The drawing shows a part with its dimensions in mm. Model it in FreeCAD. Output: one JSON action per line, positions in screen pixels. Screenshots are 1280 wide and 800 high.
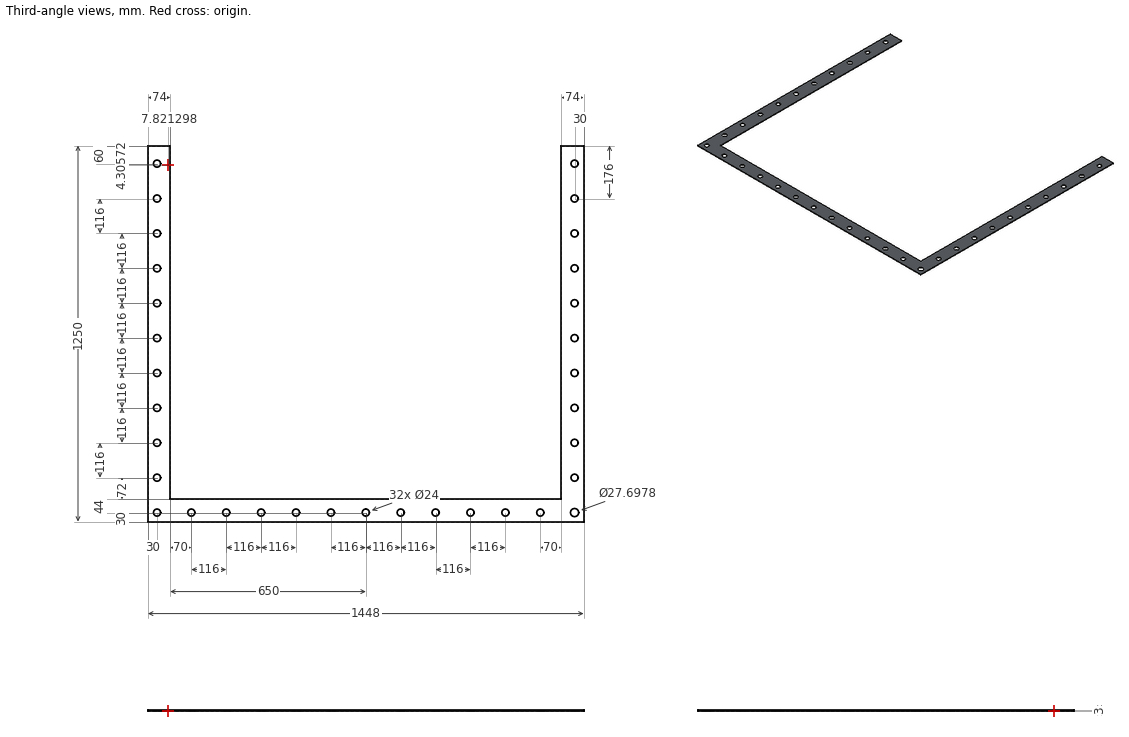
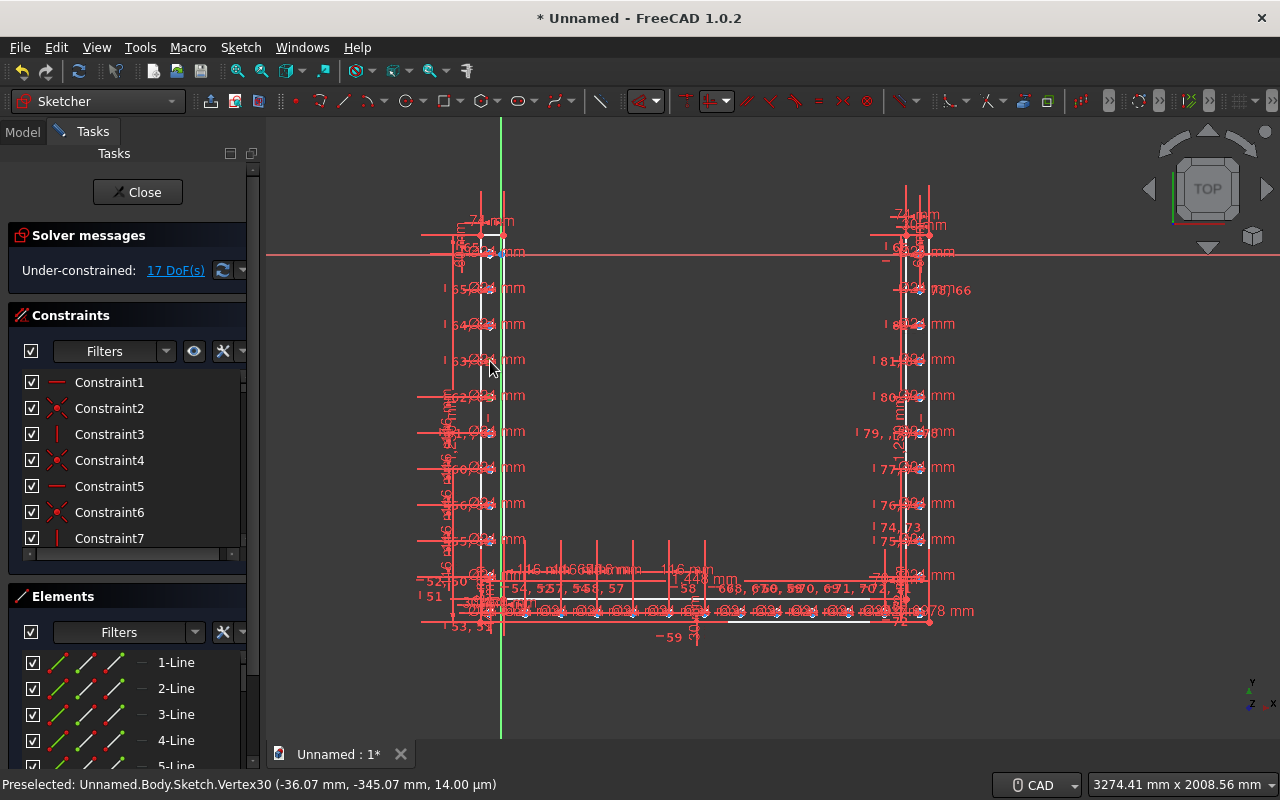
{"action": "left_click", "coordinate": [658, 102]}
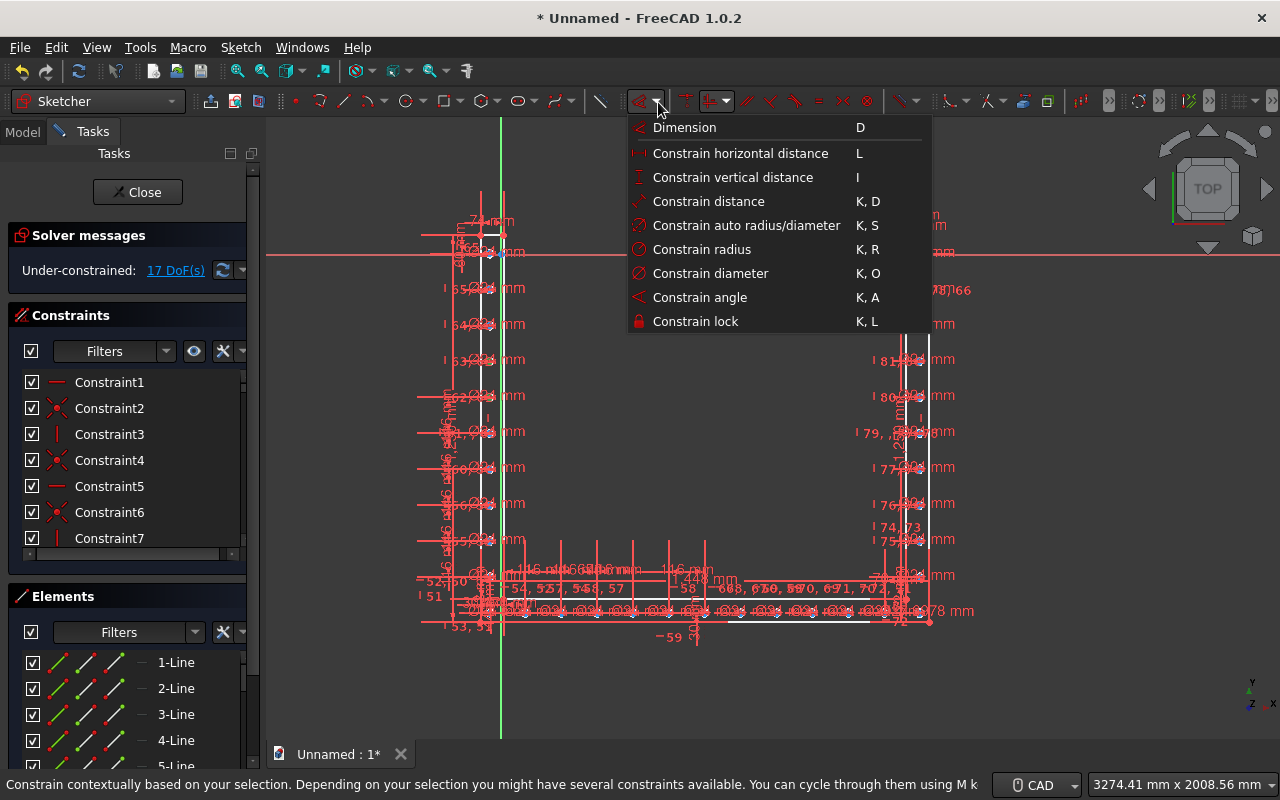
{"action": "left_click", "coordinate": [780, 177]}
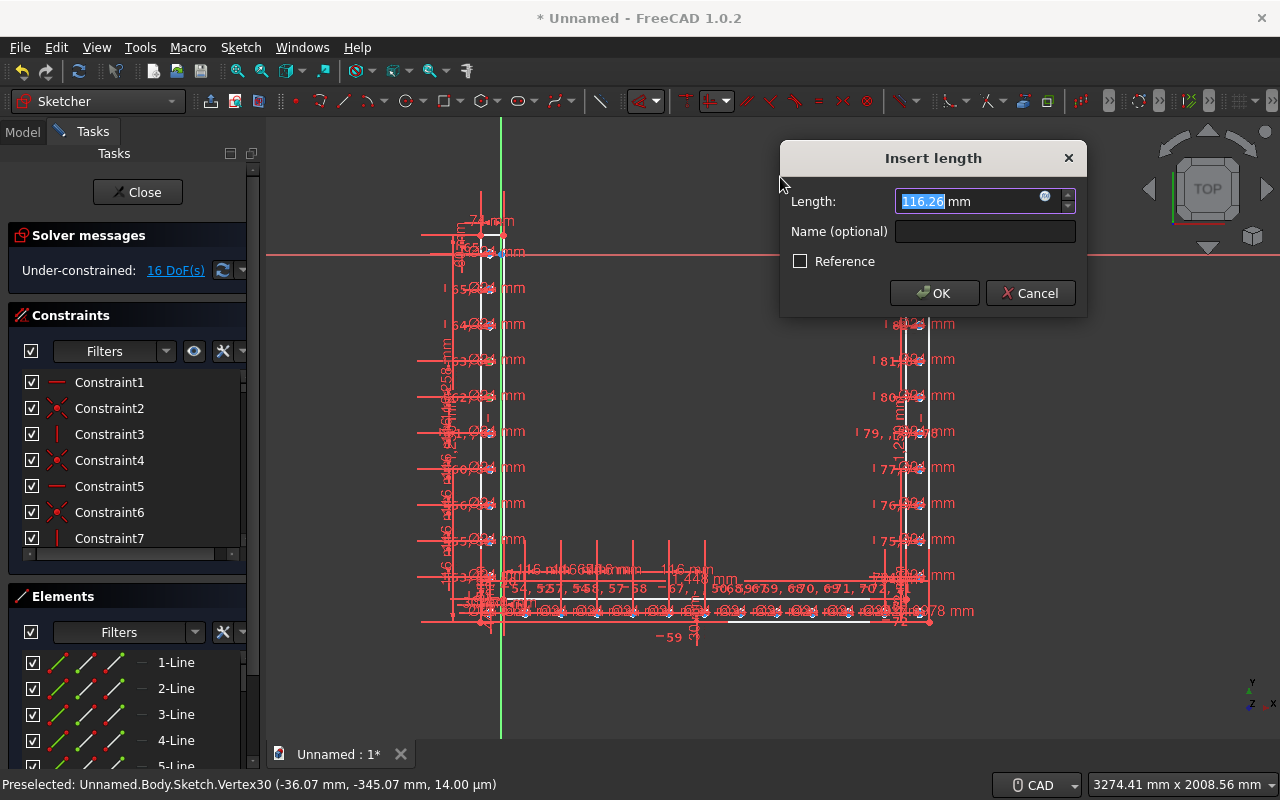
{"action": "type", "text": "116"}
{"action": "key", "text": "Return"}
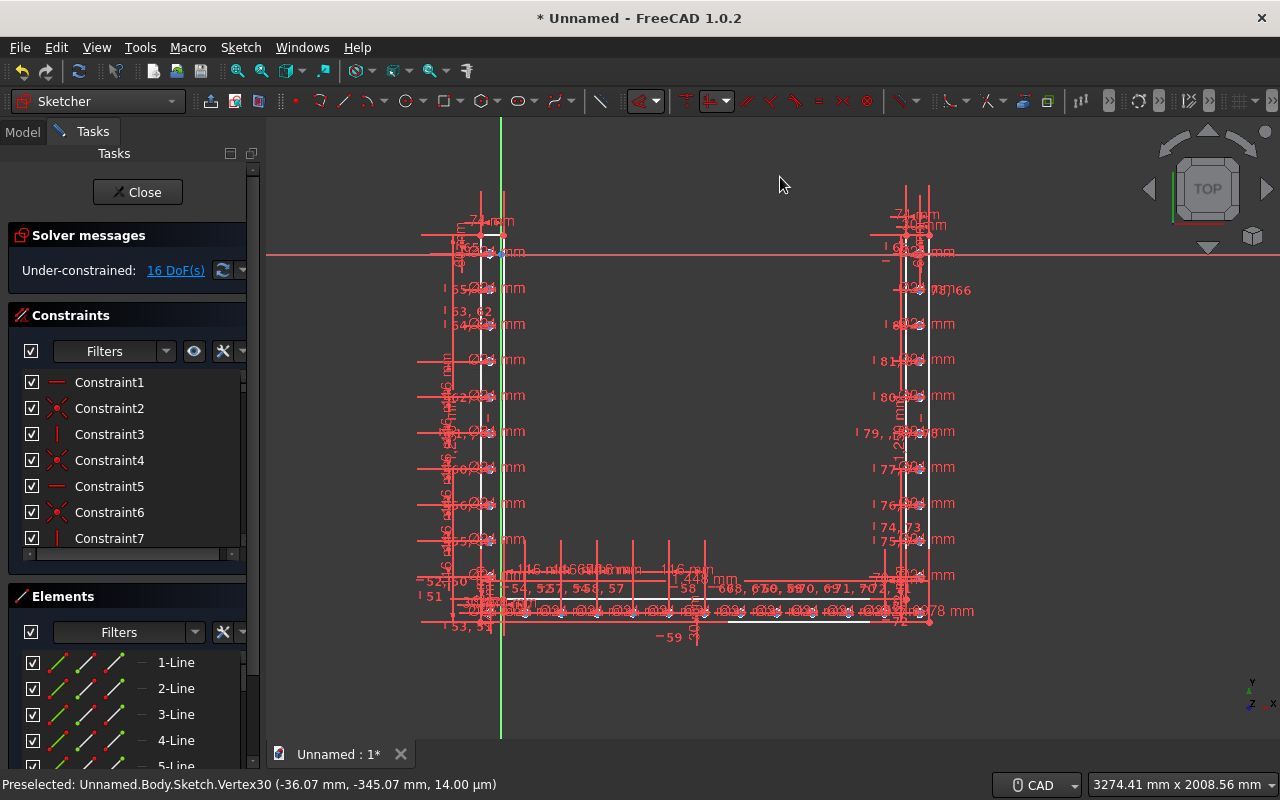
{"action": "left_click", "coordinate": [490, 362]}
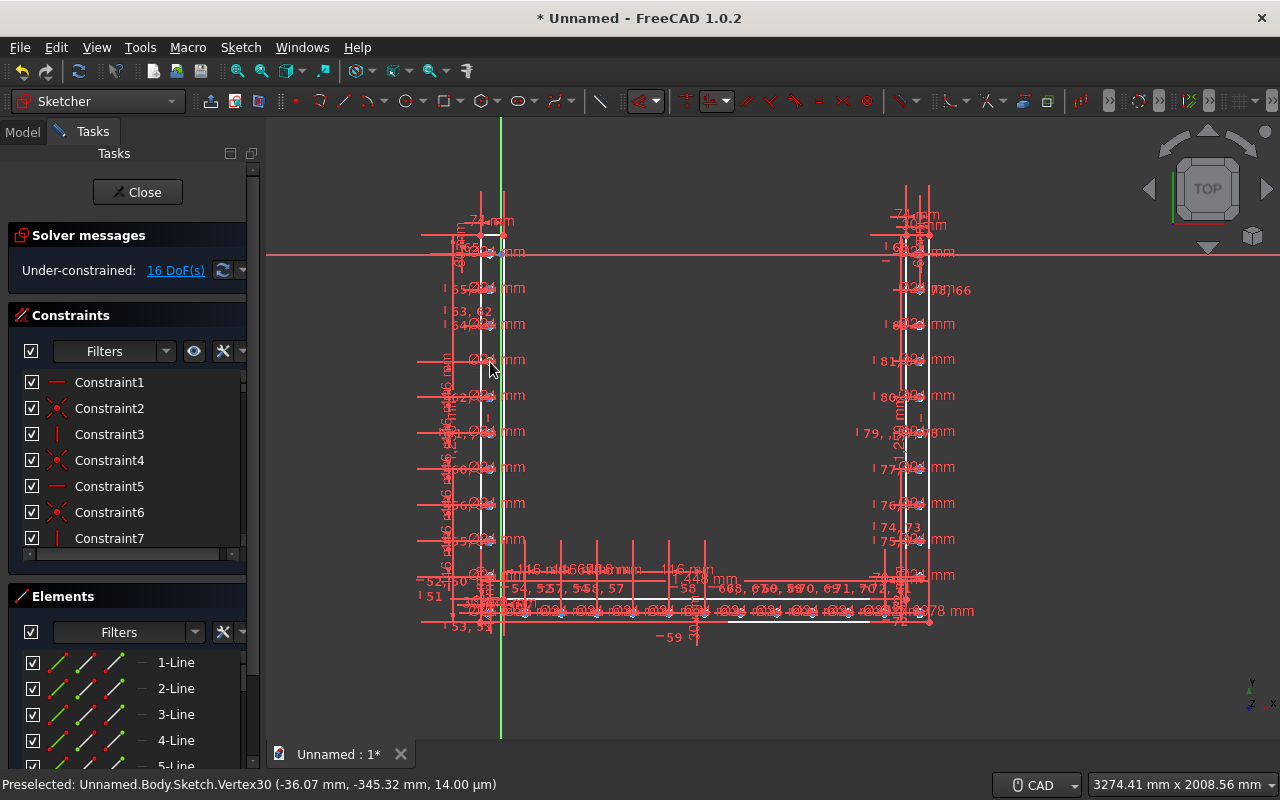
{"action": "left_click", "coordinate": [490, 326]}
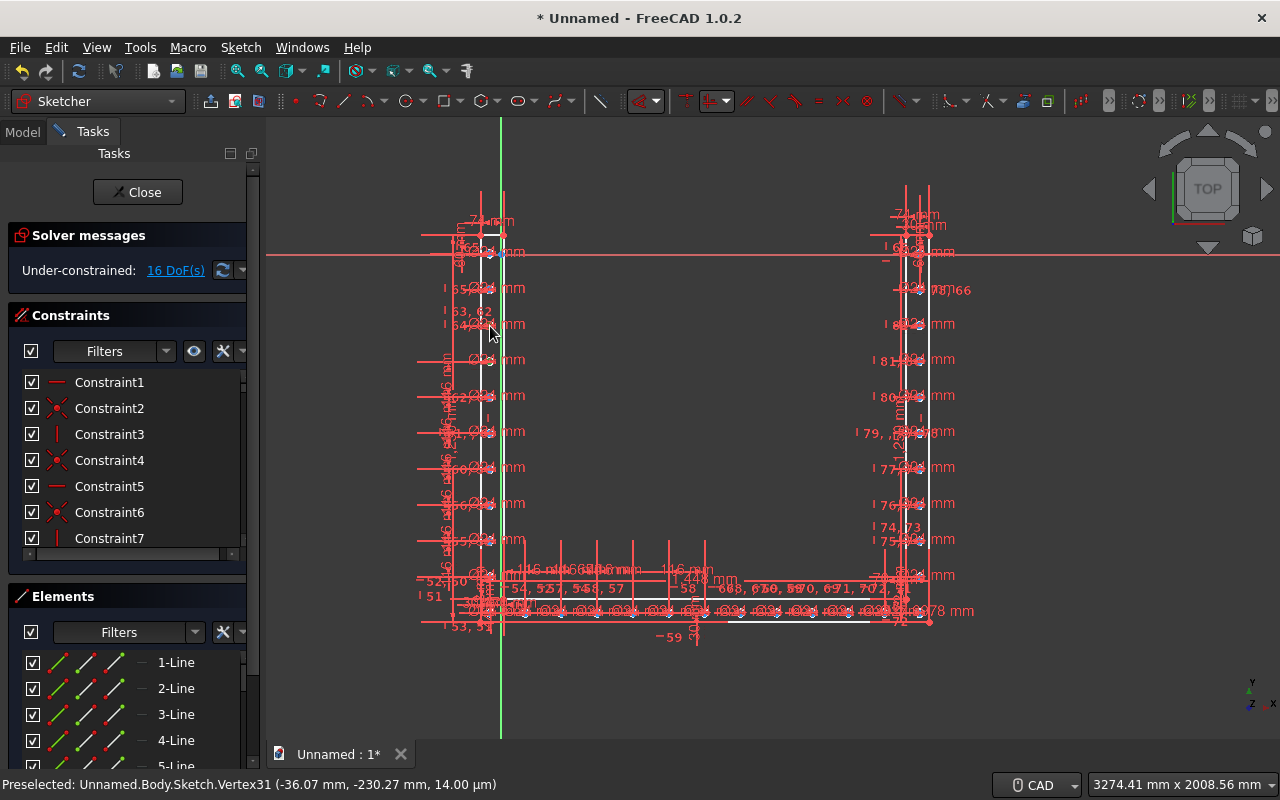
{"action": "left_click", "coordinate": [658, 102]}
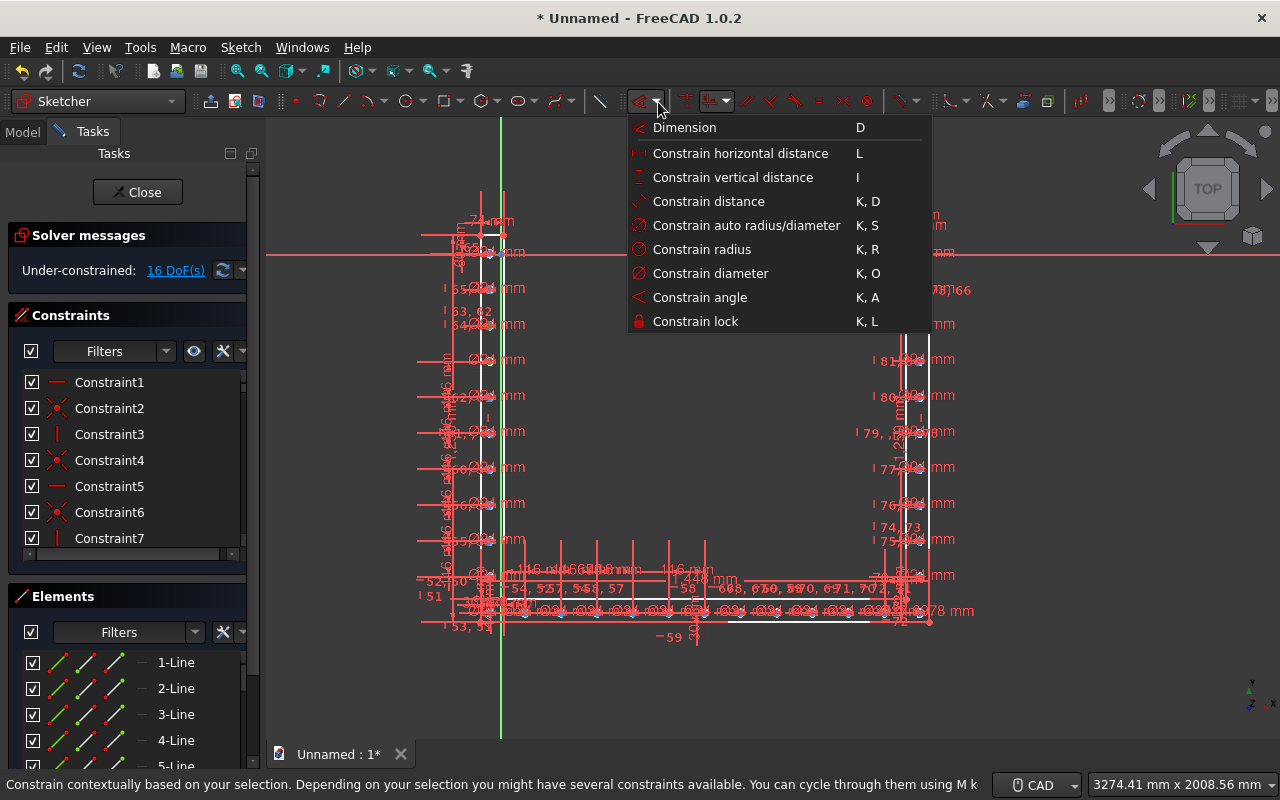
{"action": "left_click", "coordinate": [780, 177]}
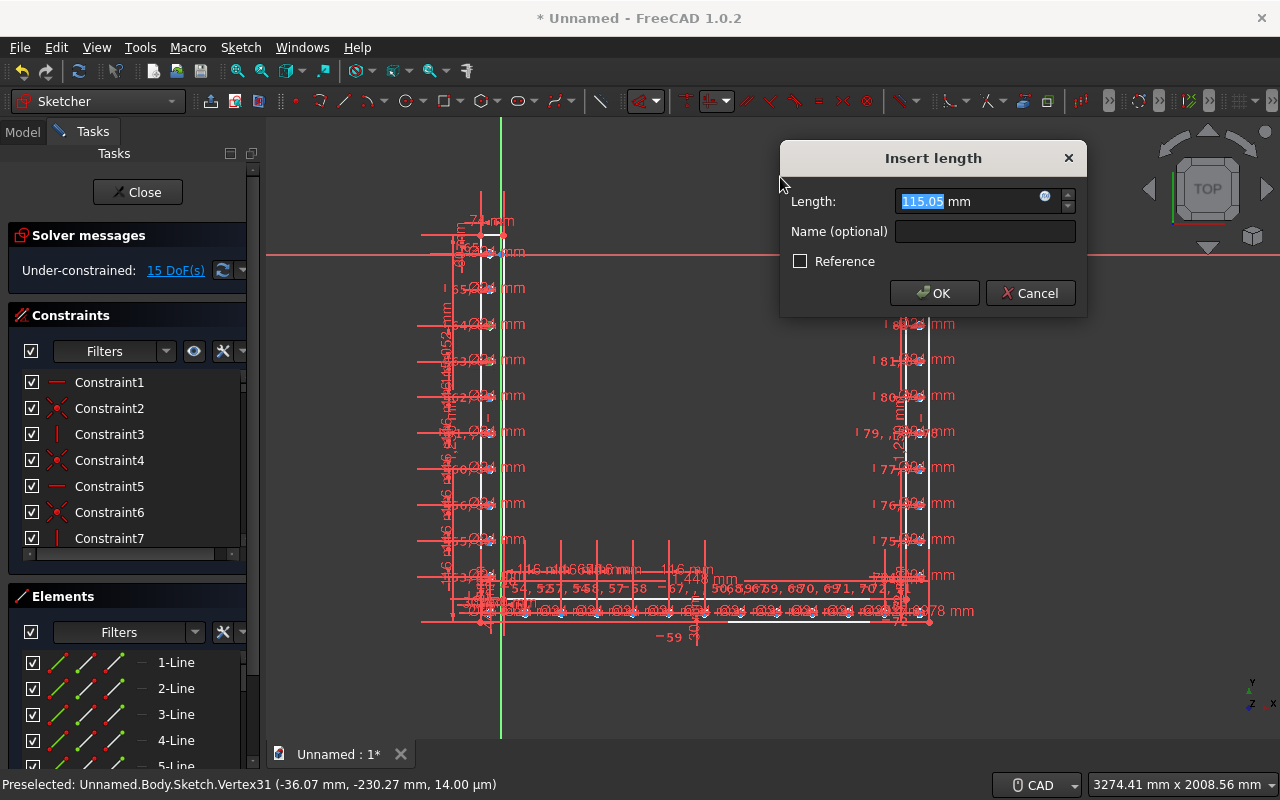
{"action": "type", "text": "116"}
{"action": "key", "text": "Return"}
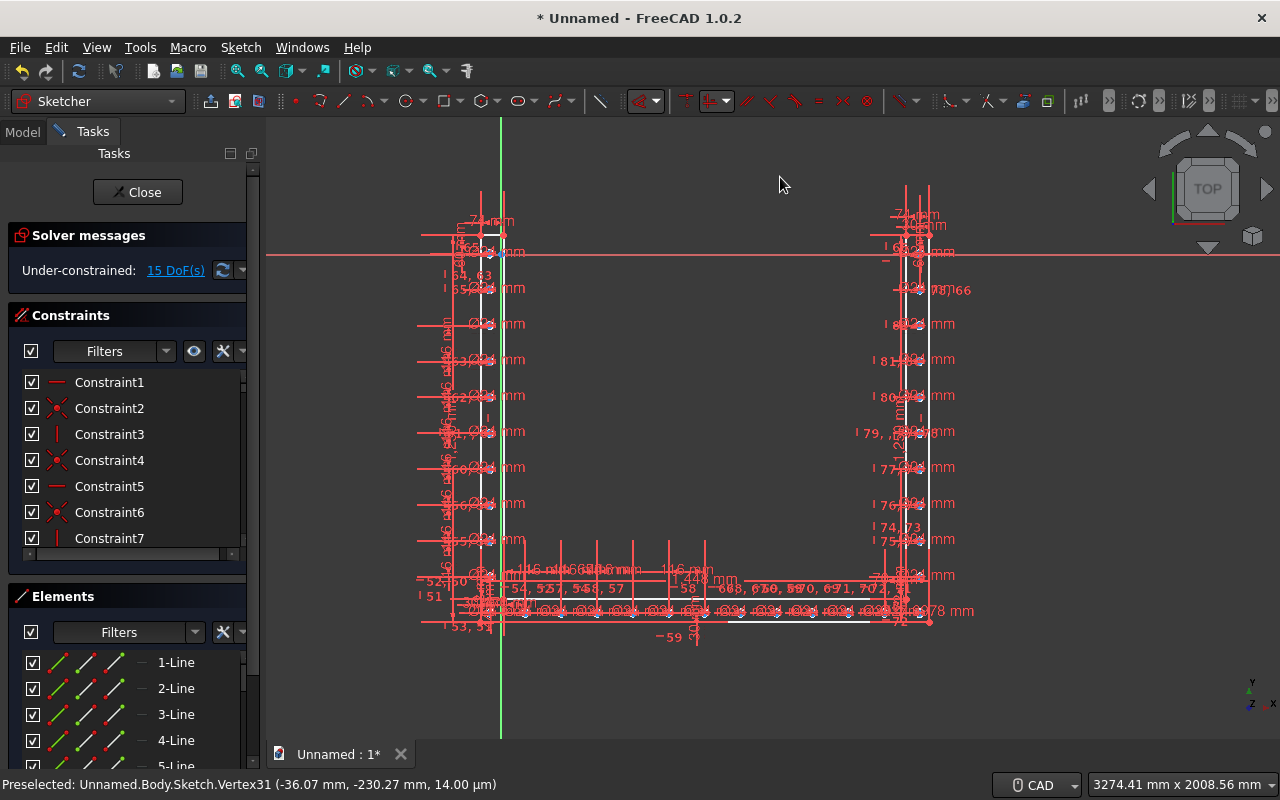
{"action": "left_click", "coordinate": [490, 326]}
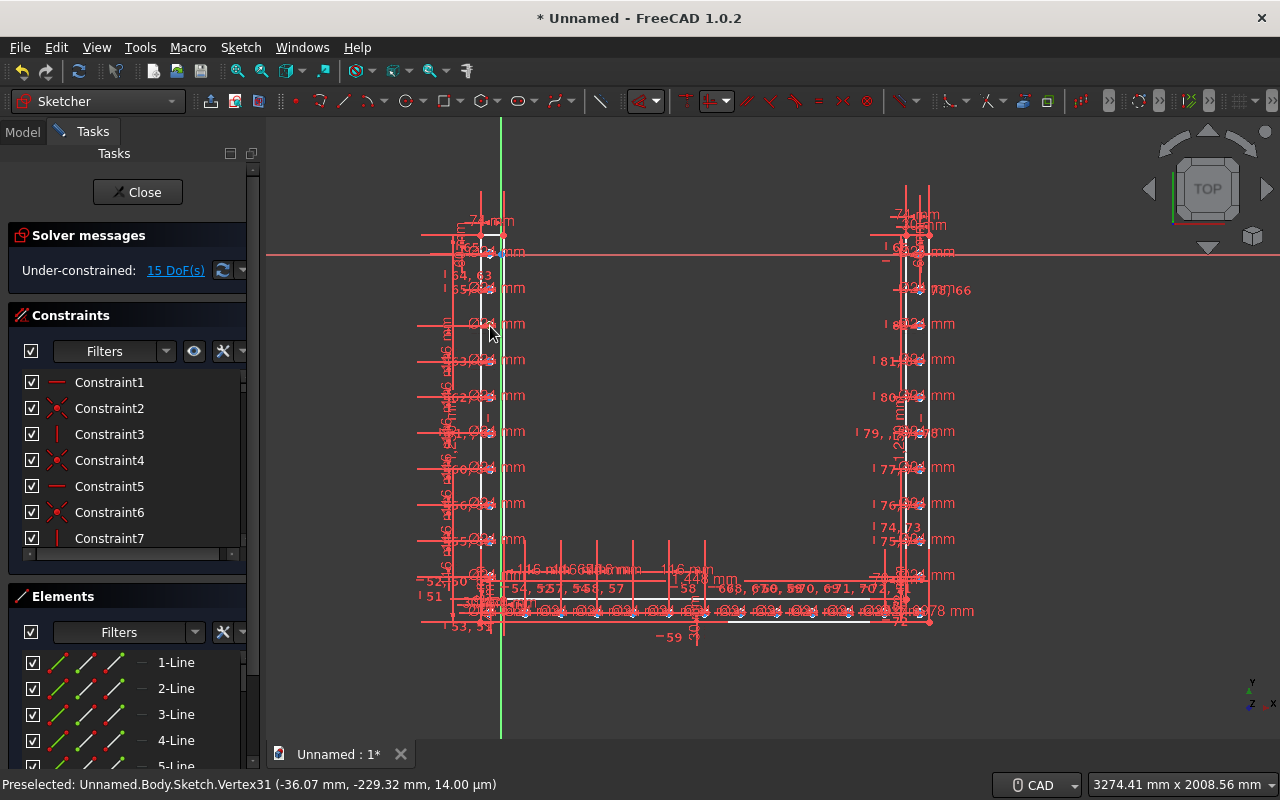
{"action": "left_click", "coordinate": [490, 290]}